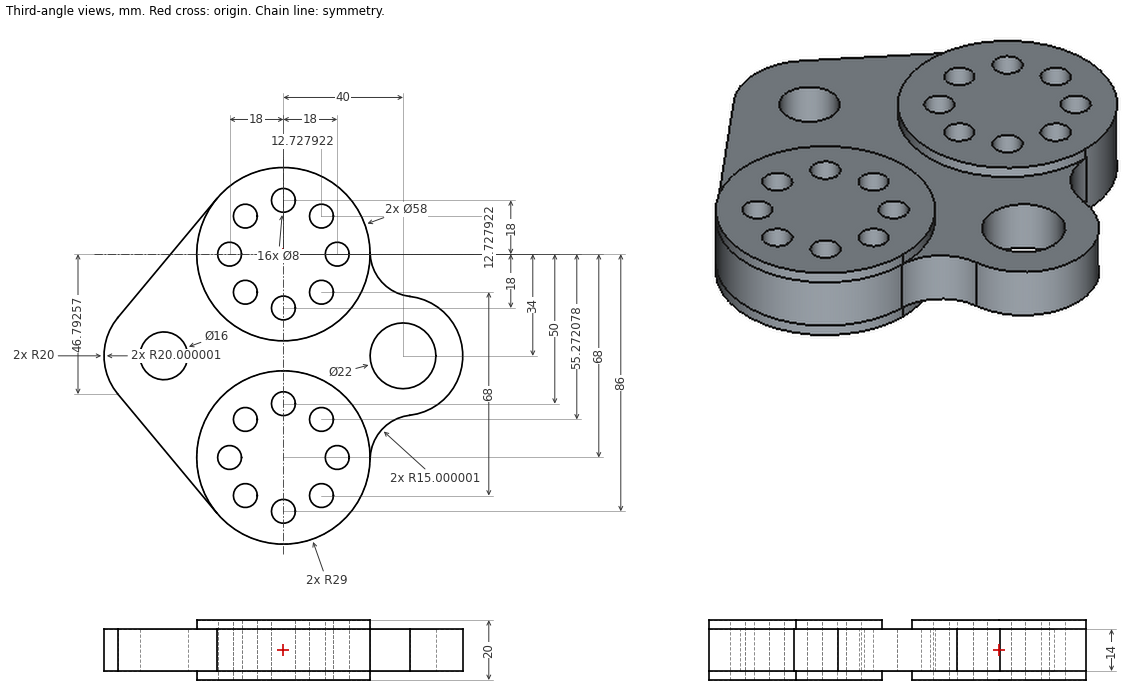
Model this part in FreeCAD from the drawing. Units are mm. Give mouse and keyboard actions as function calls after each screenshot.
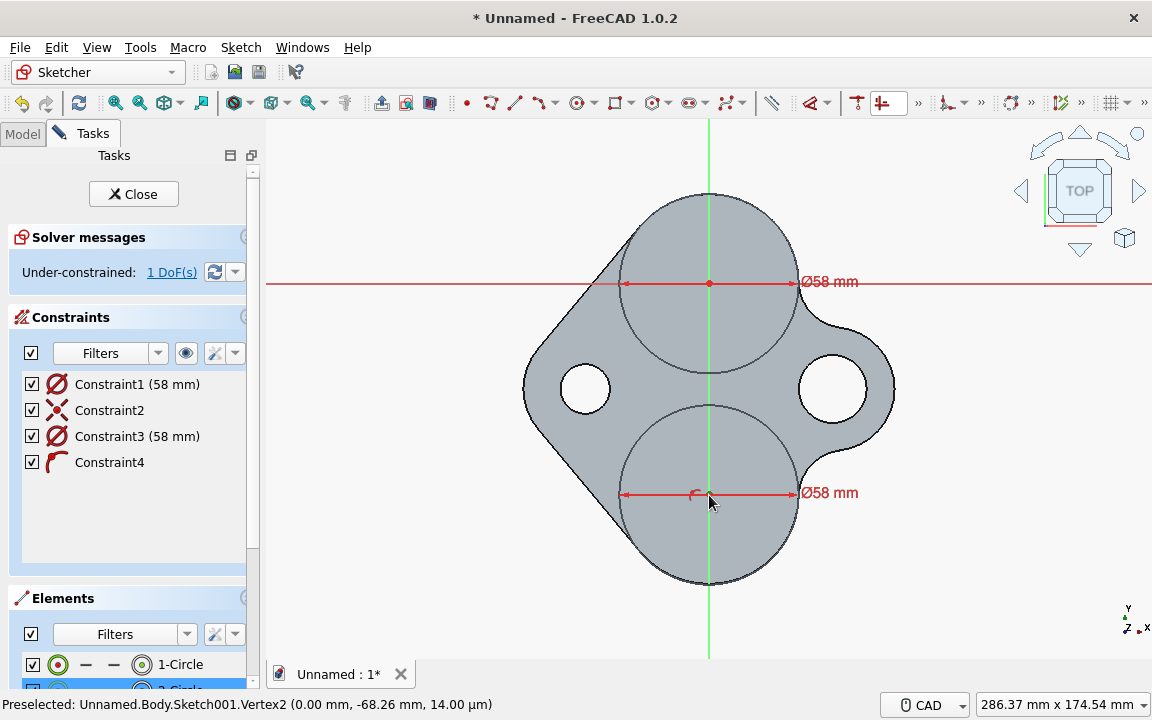
click(830, 104)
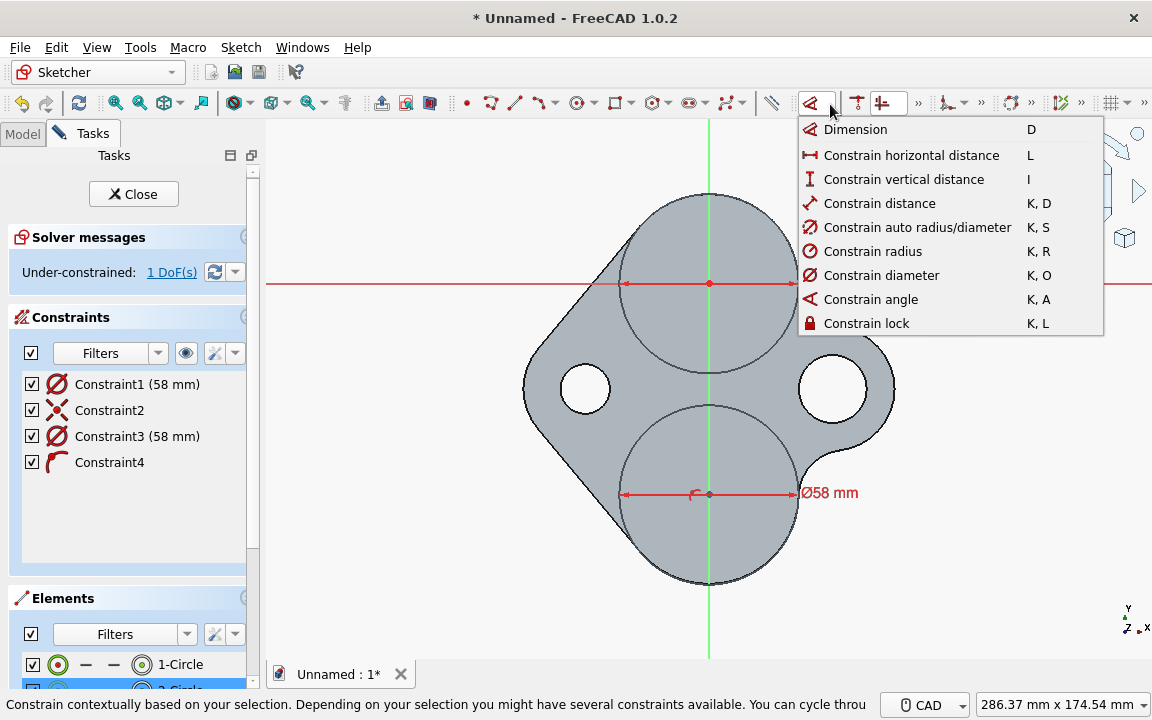
click(951, 179)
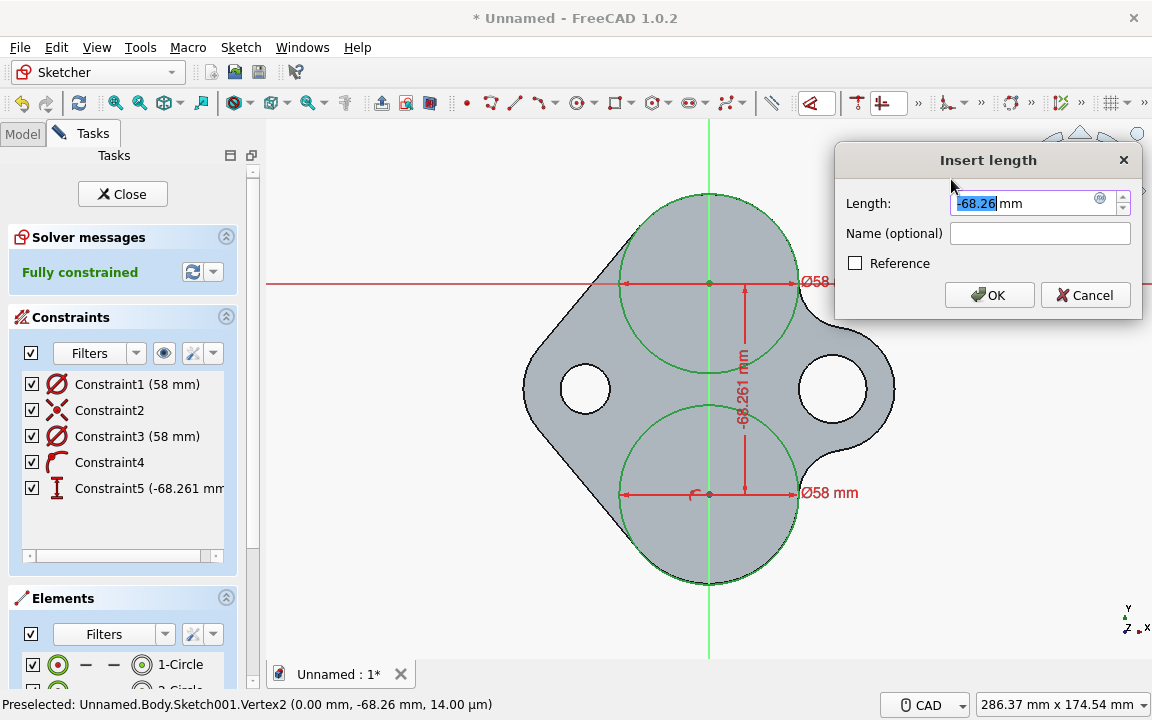
text(-68)
key(Return)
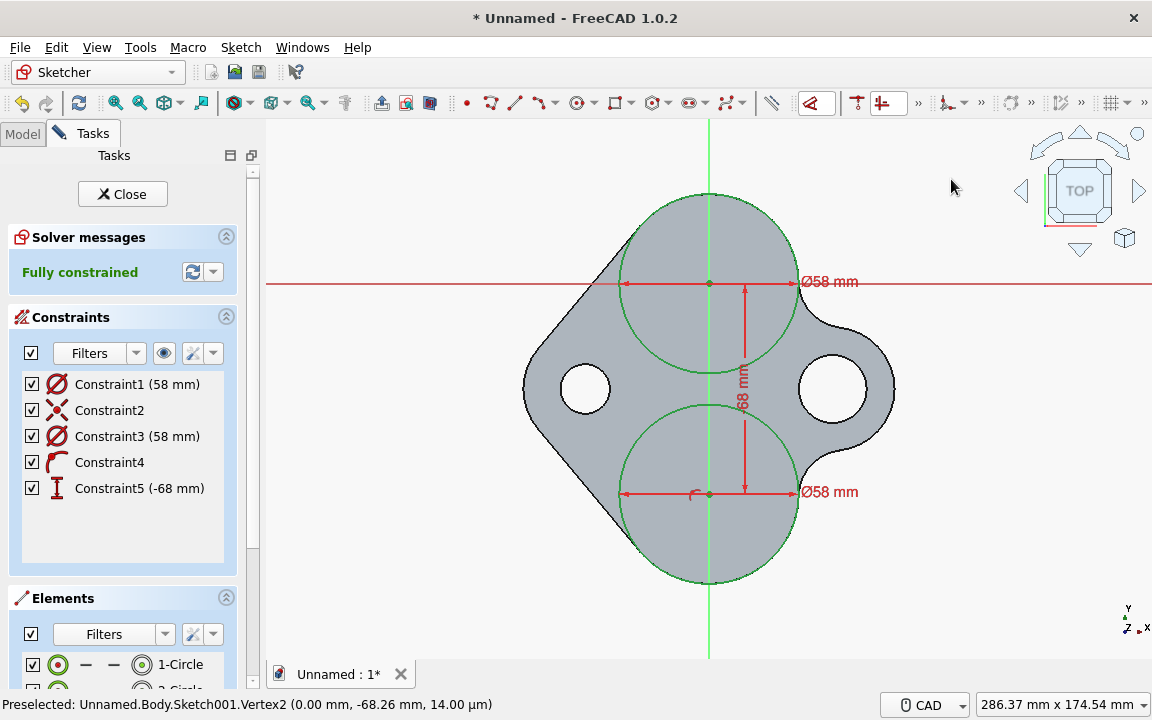
click(123, 194)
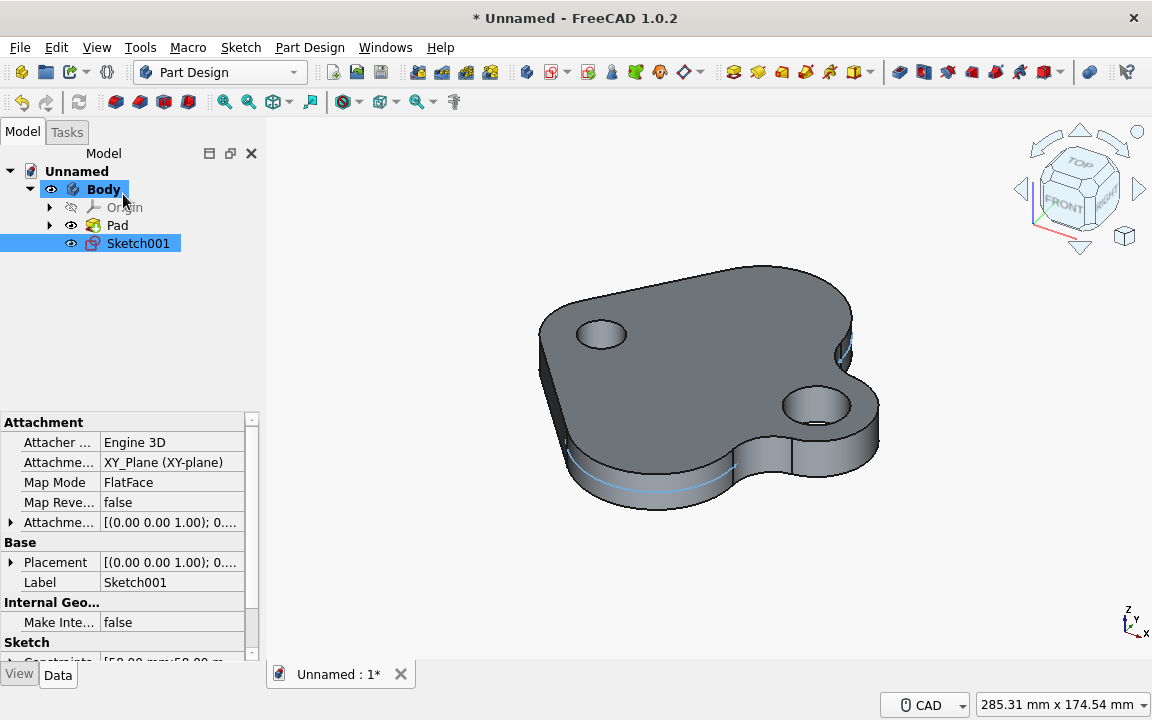
click(734, 72)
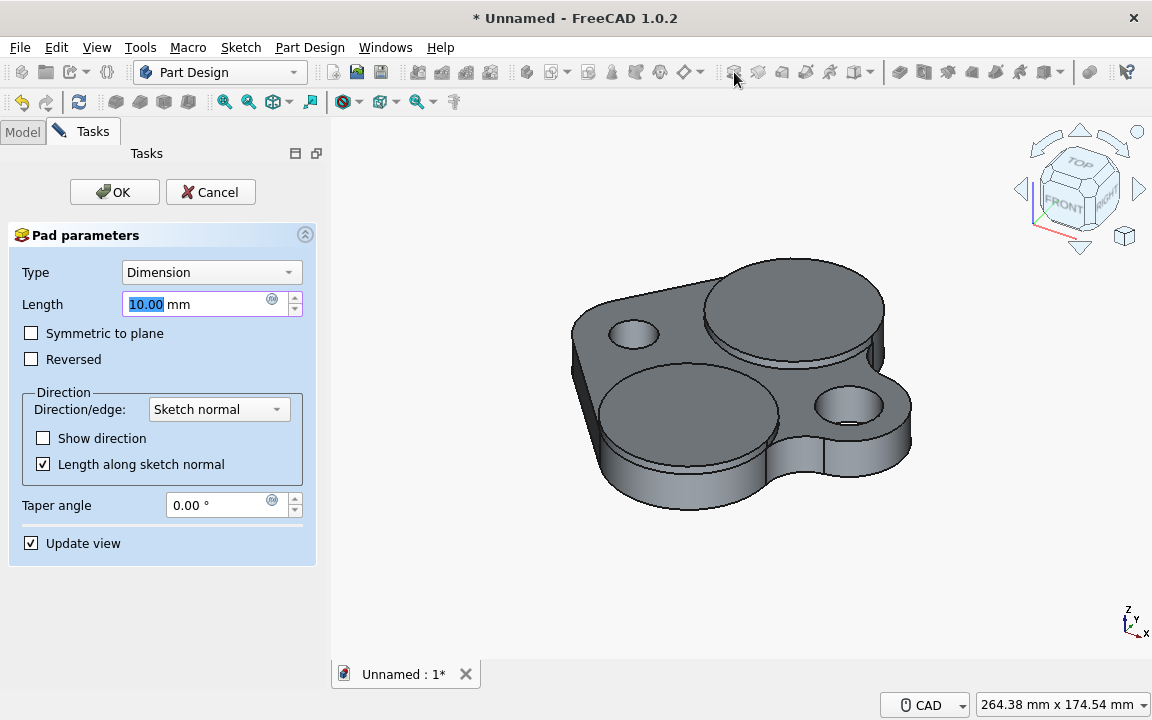
text(20)
key(Tab)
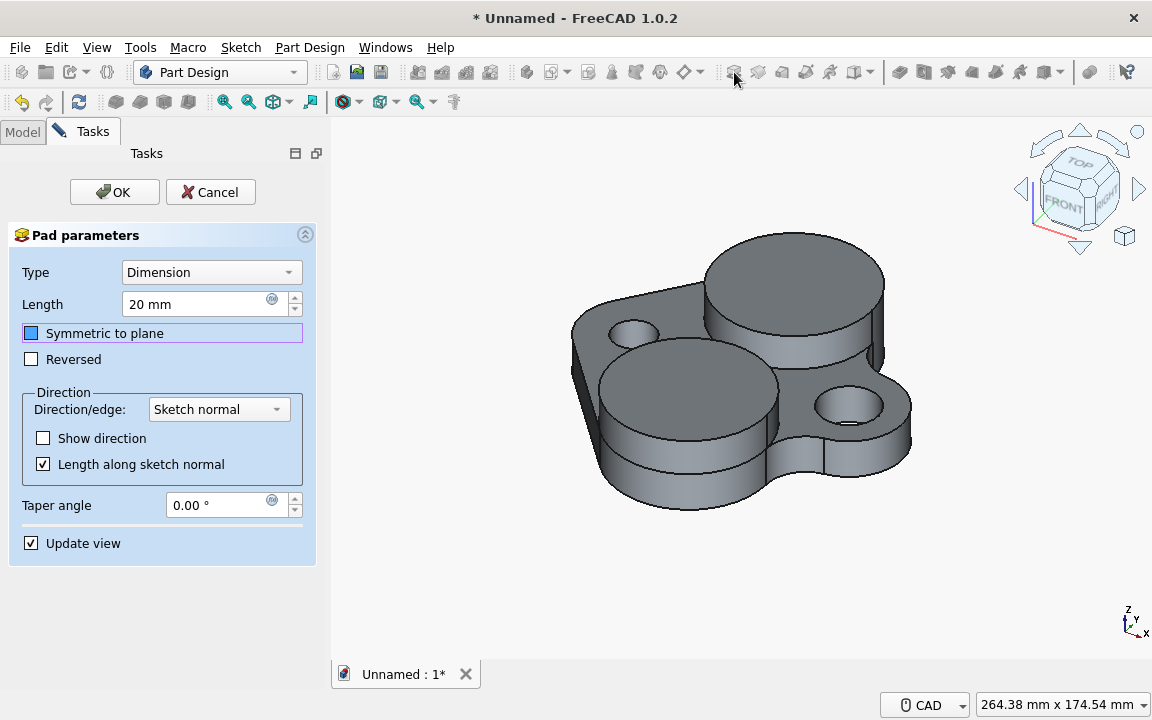
click(30, 333)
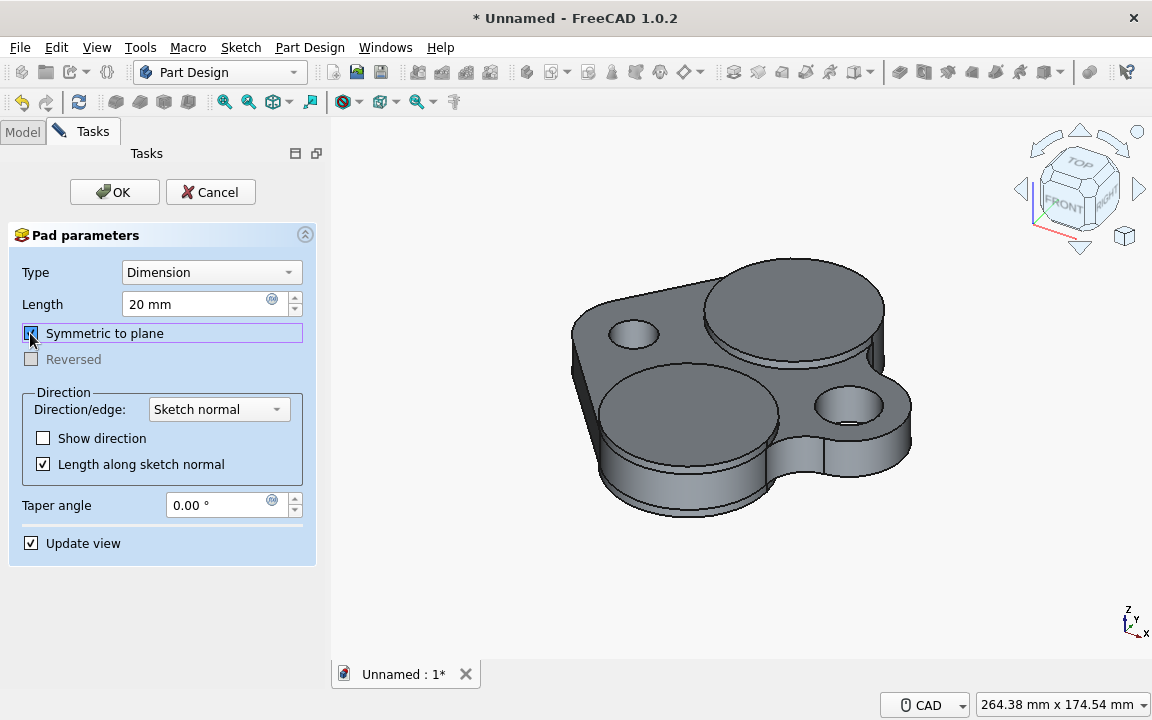
click(115, 192)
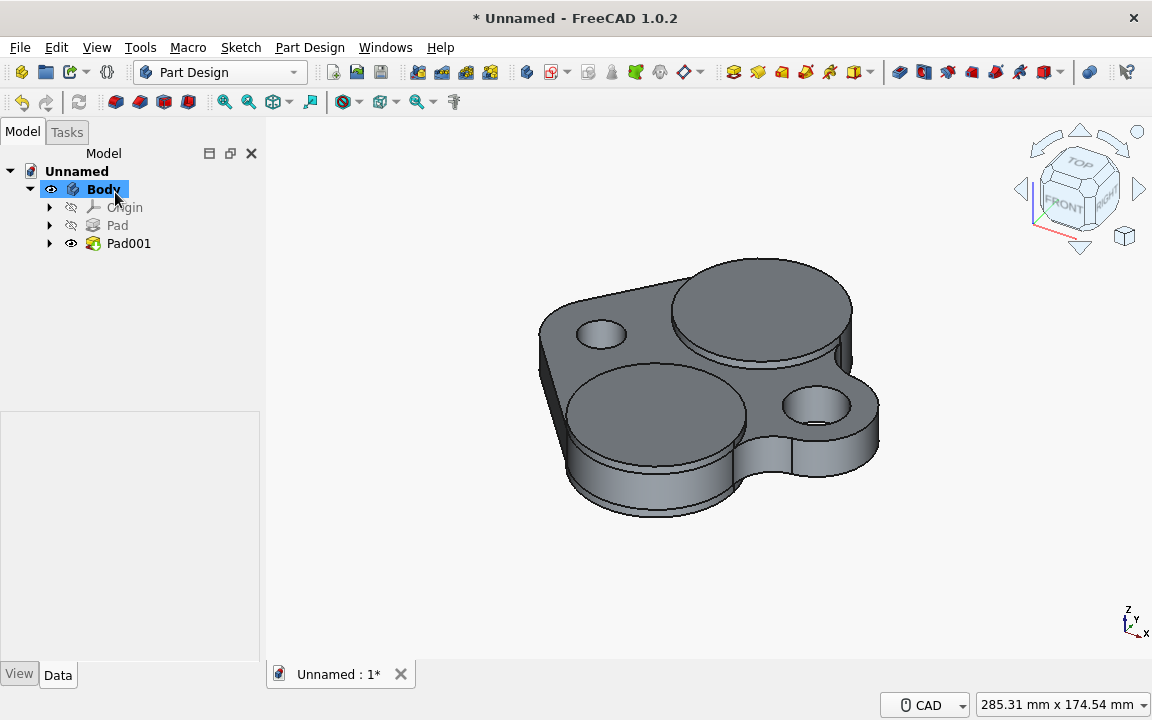
click(762, 309)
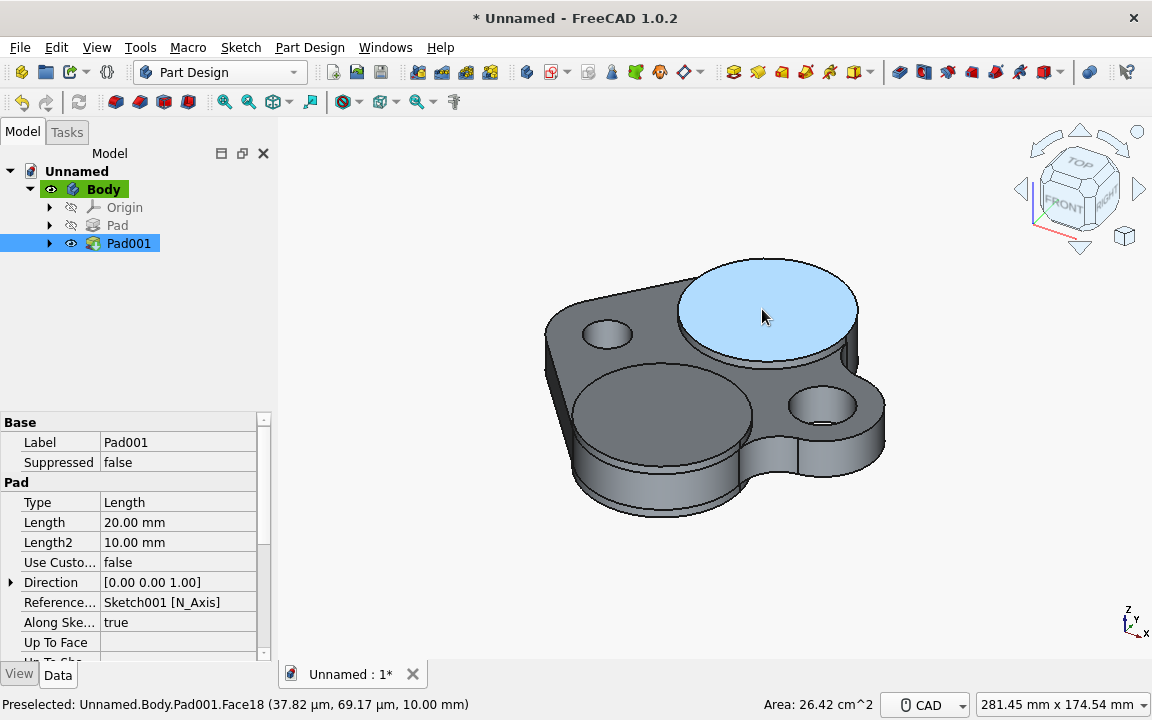
click(552, 72)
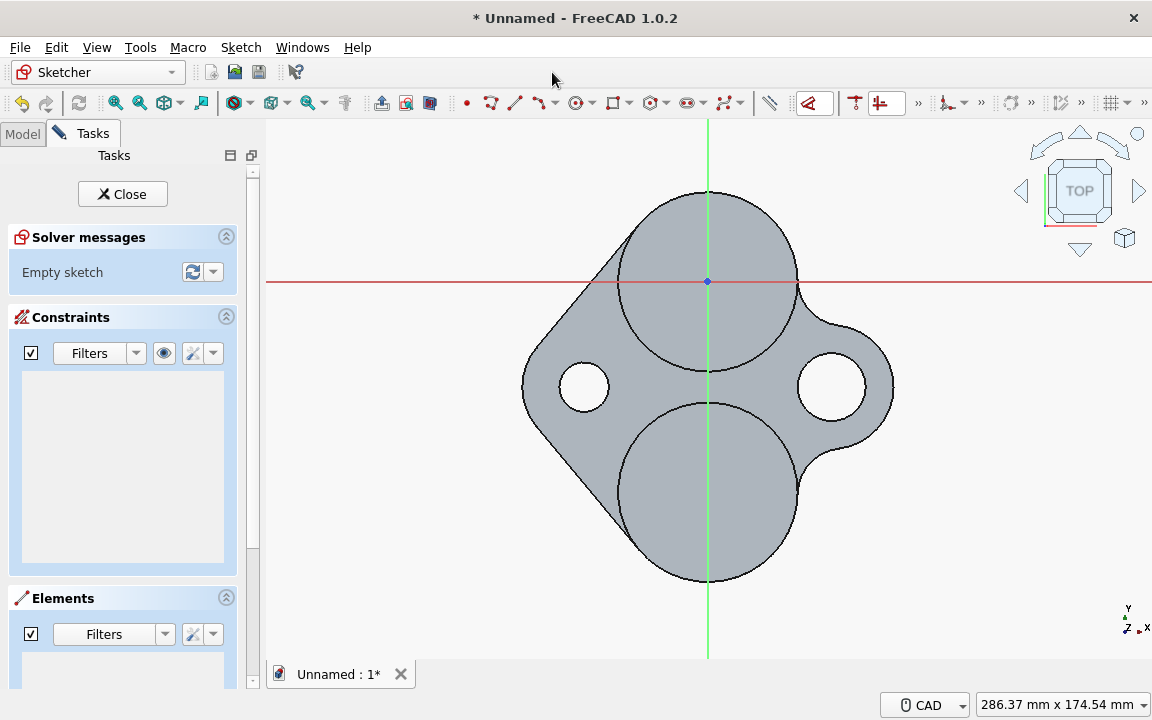
key(g)
key(c)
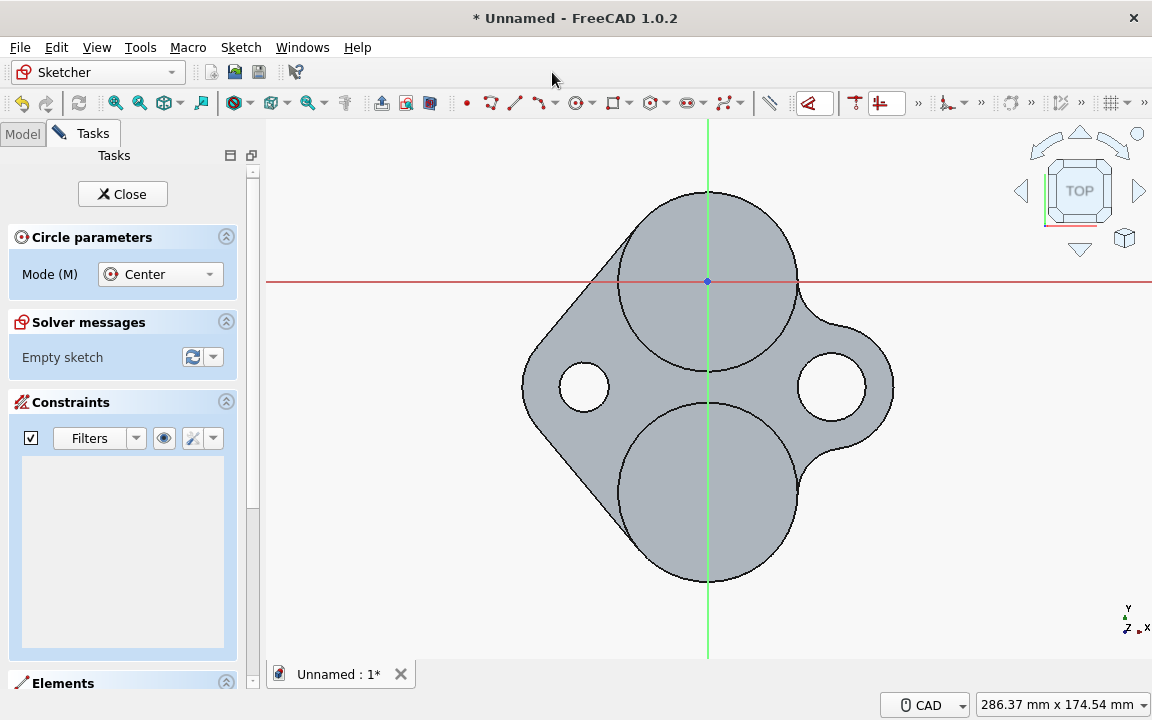
scroll(708, 226, up, 4)